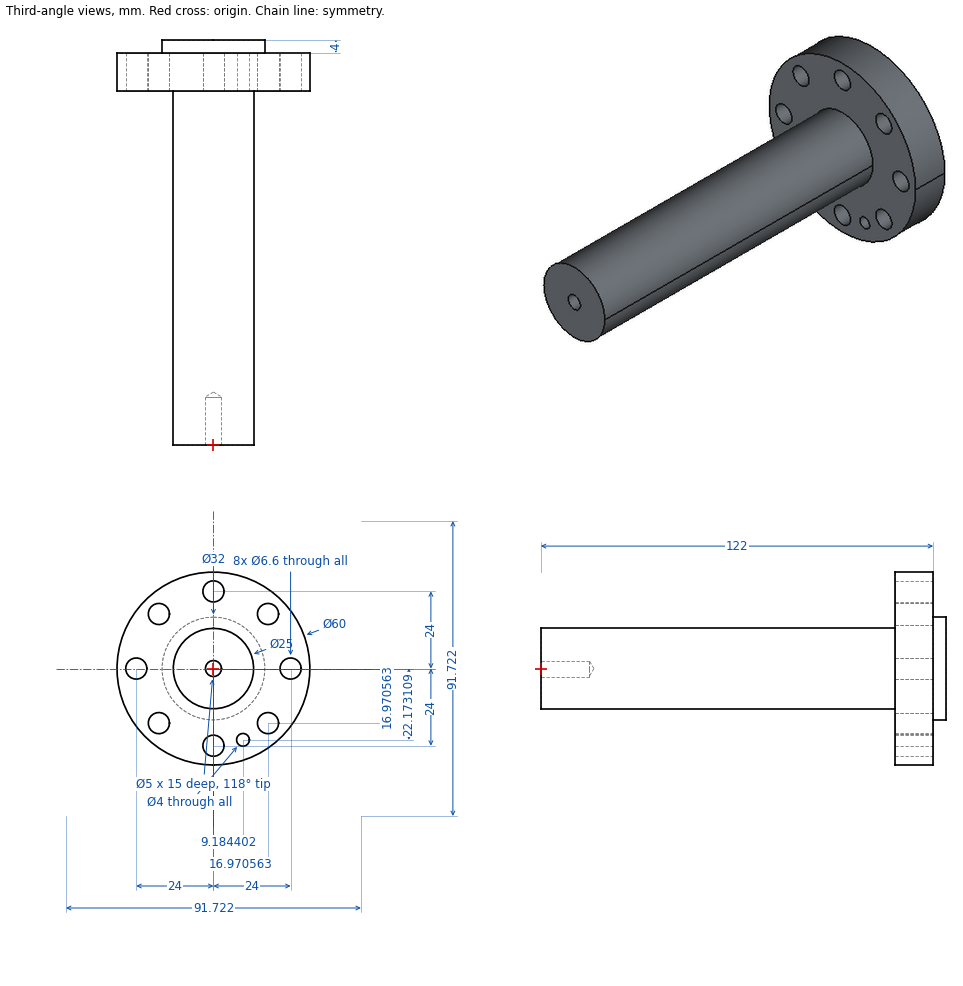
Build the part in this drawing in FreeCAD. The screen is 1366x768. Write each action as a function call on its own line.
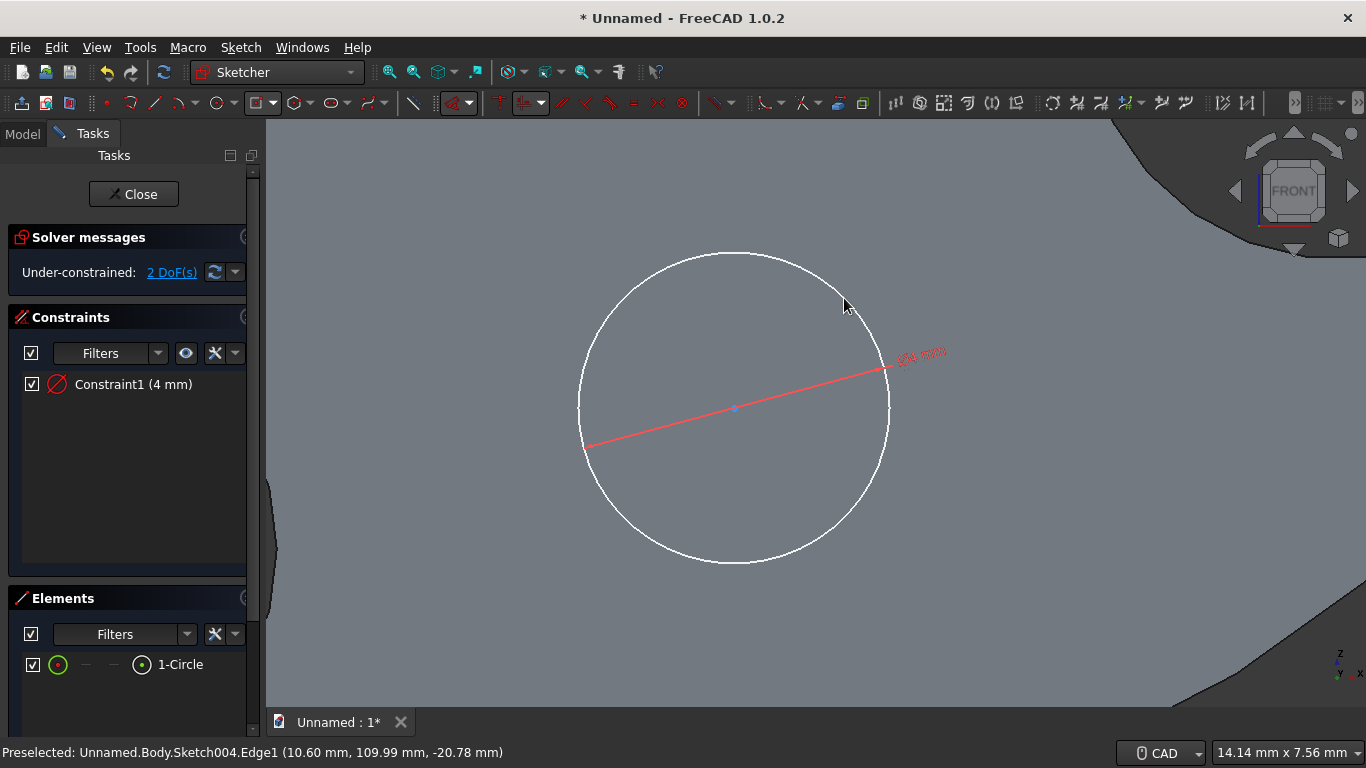
click(734, 408)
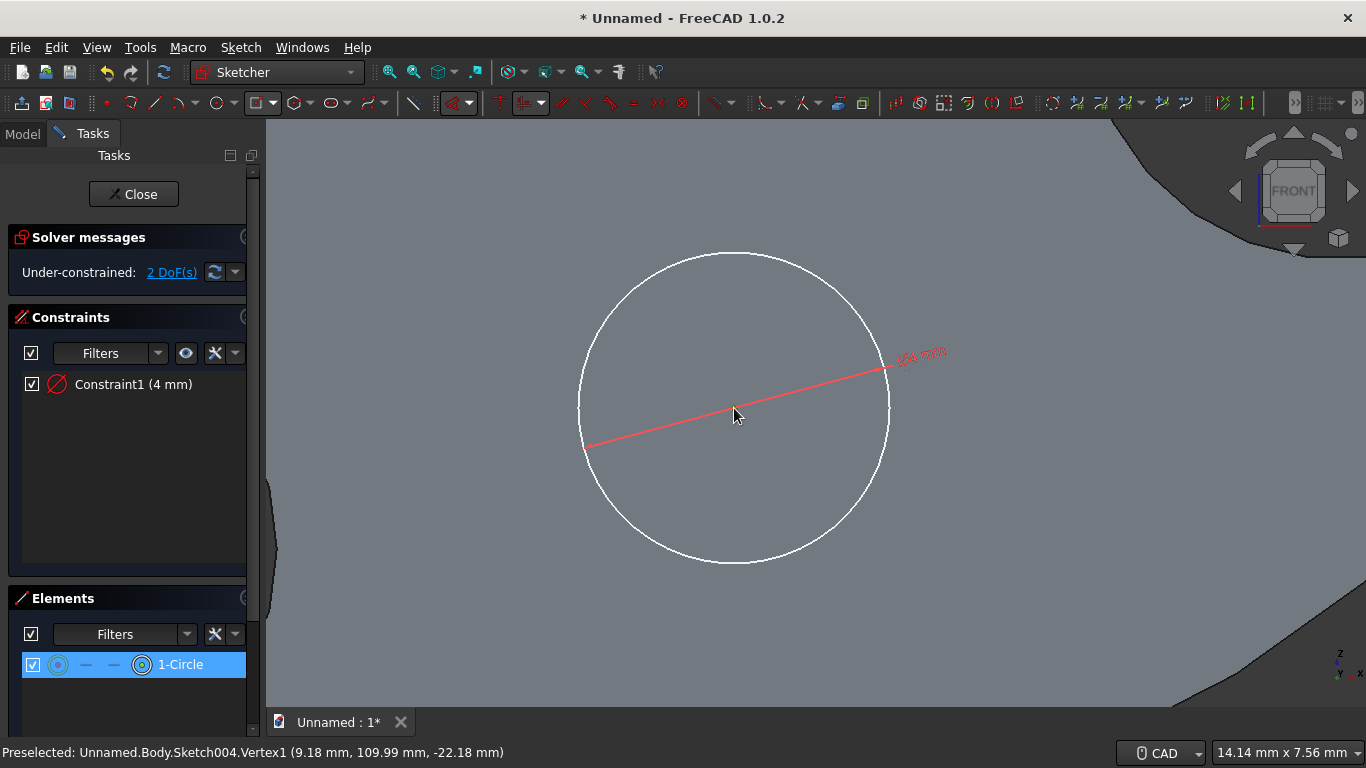
key(l)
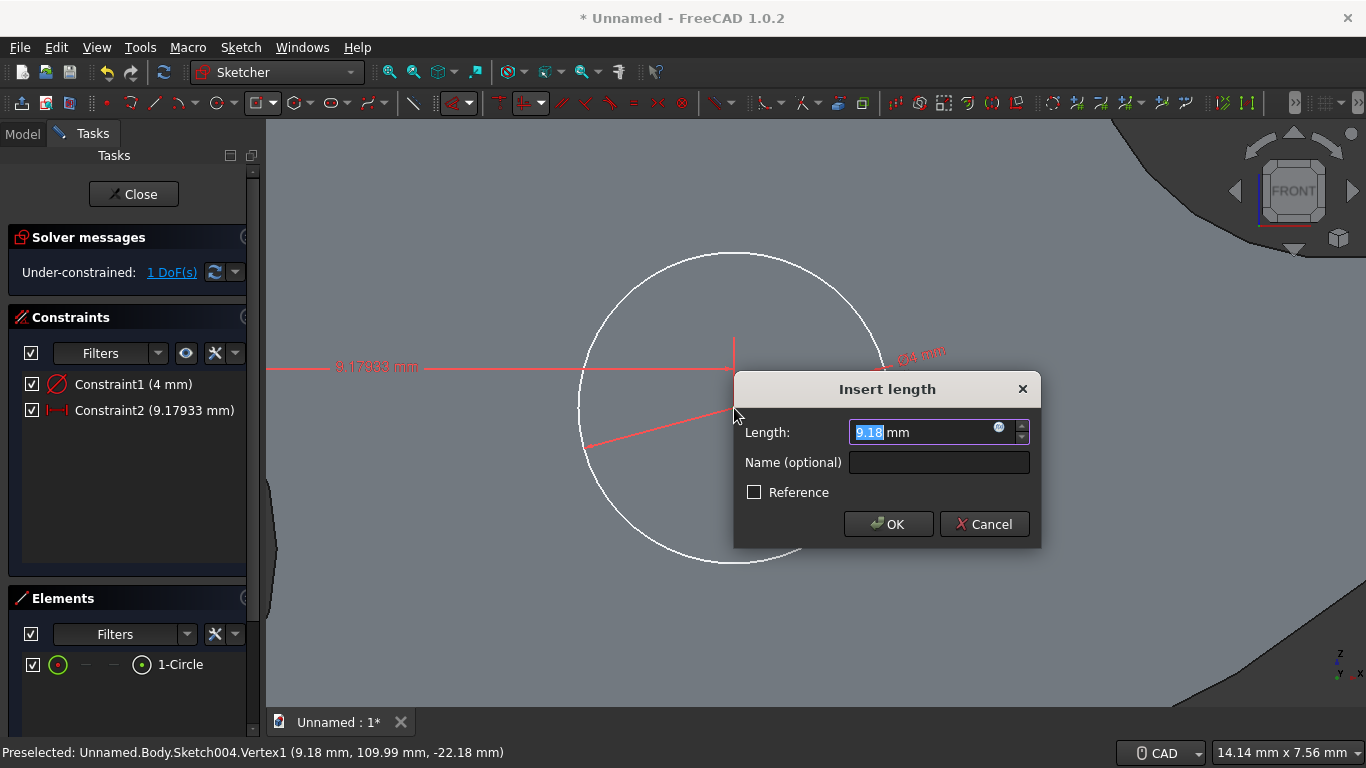
text(9.184402)
key(Return)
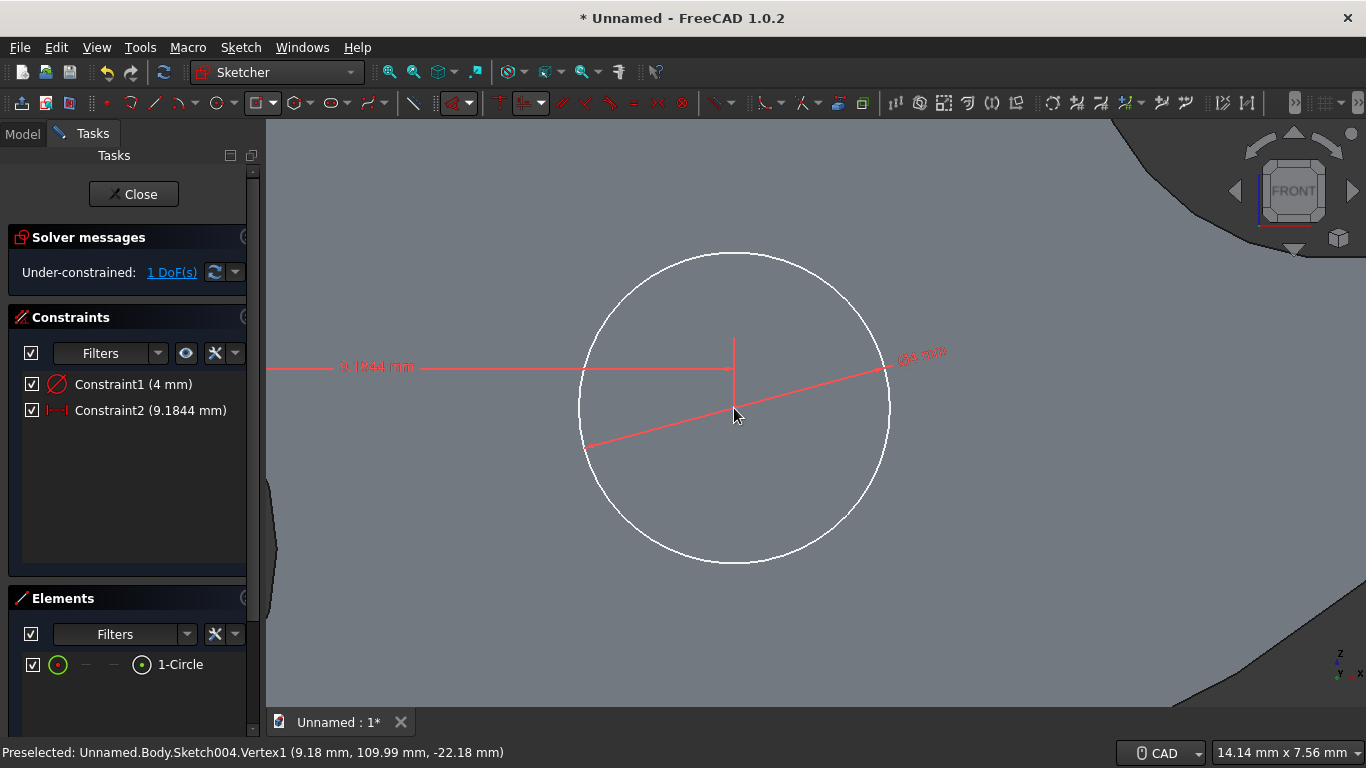
click(734, 408)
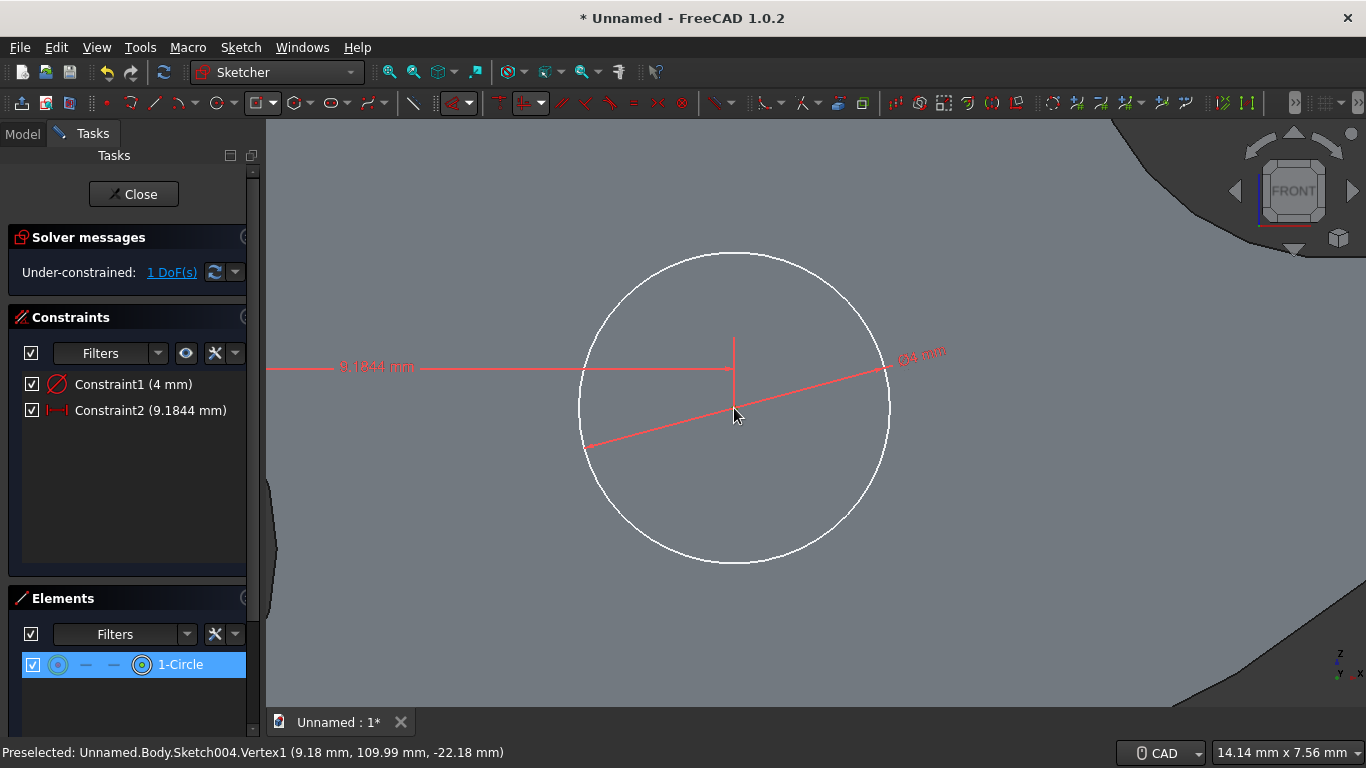
key(i)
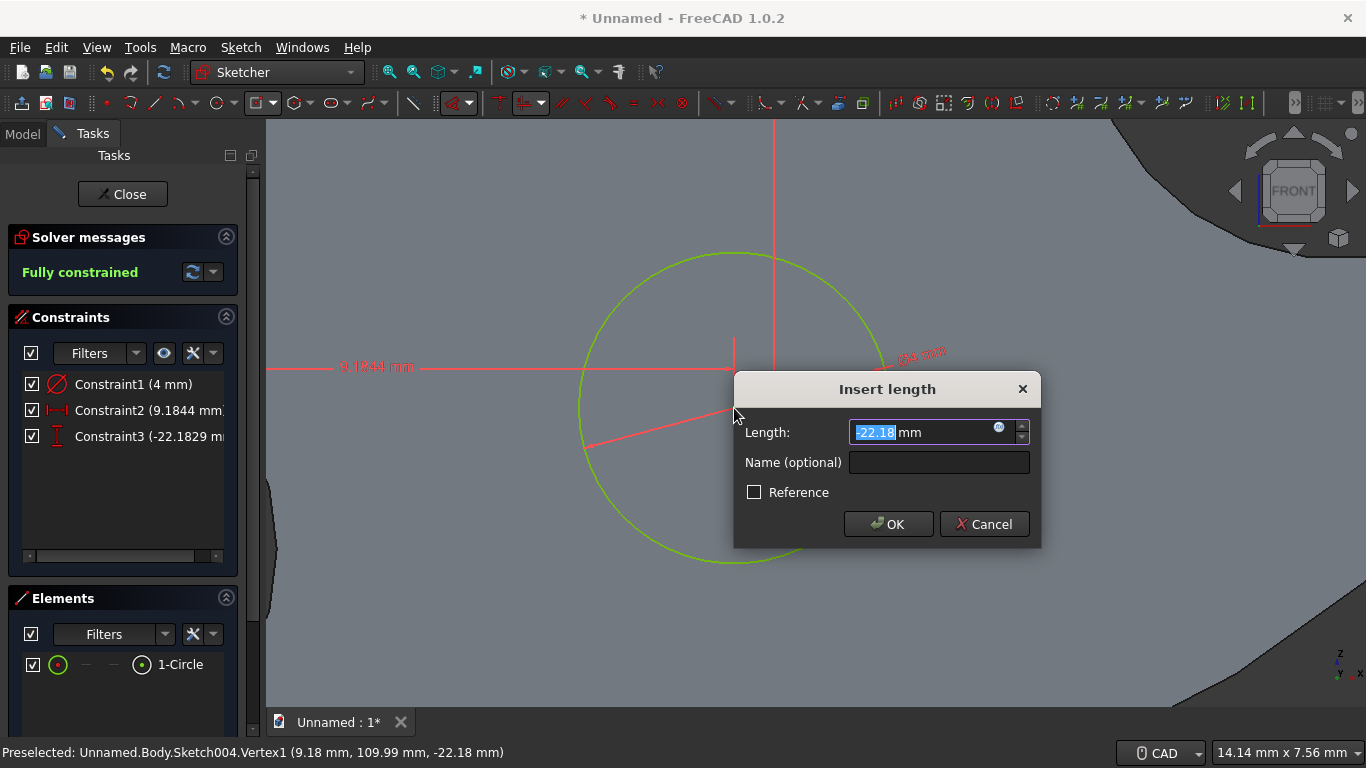
text(-22.173109)
key(Return)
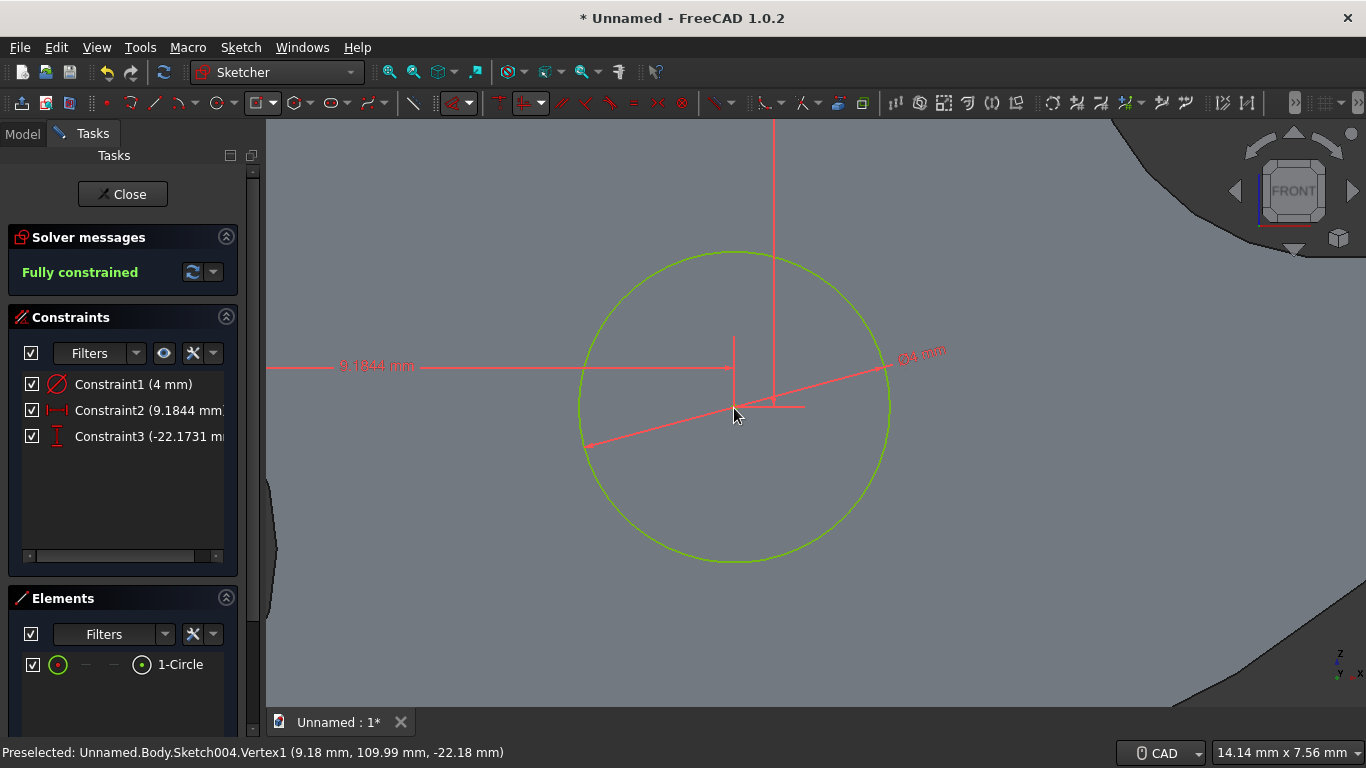
click(123, 194)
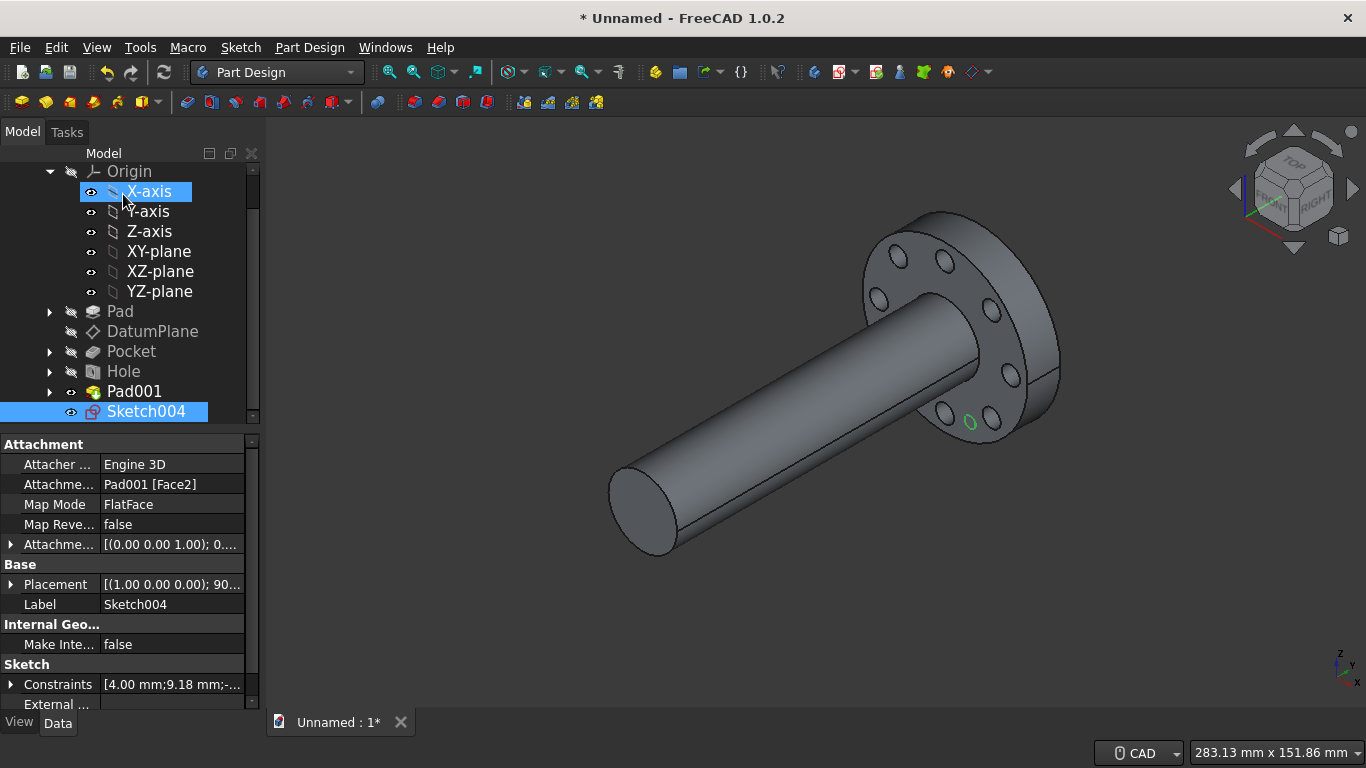
click(212, 102)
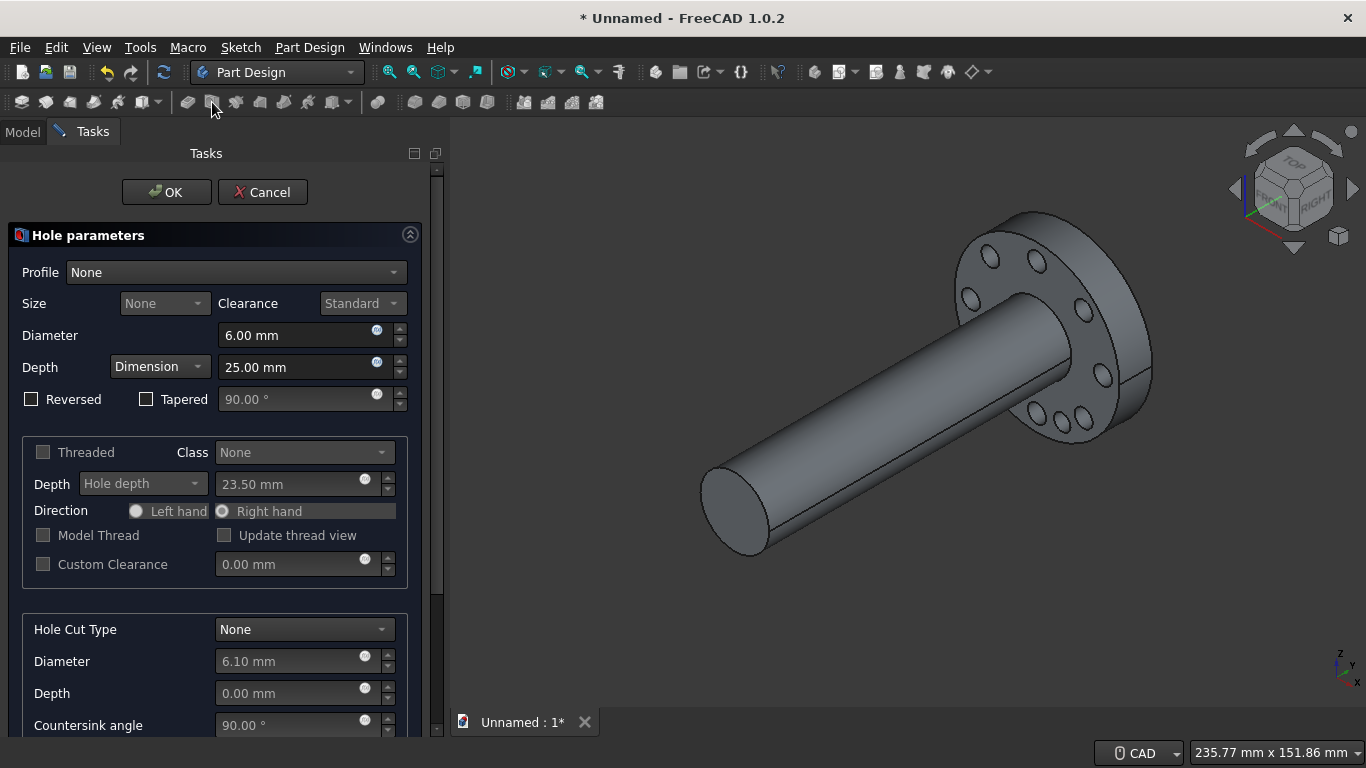
triple_click(305, 335)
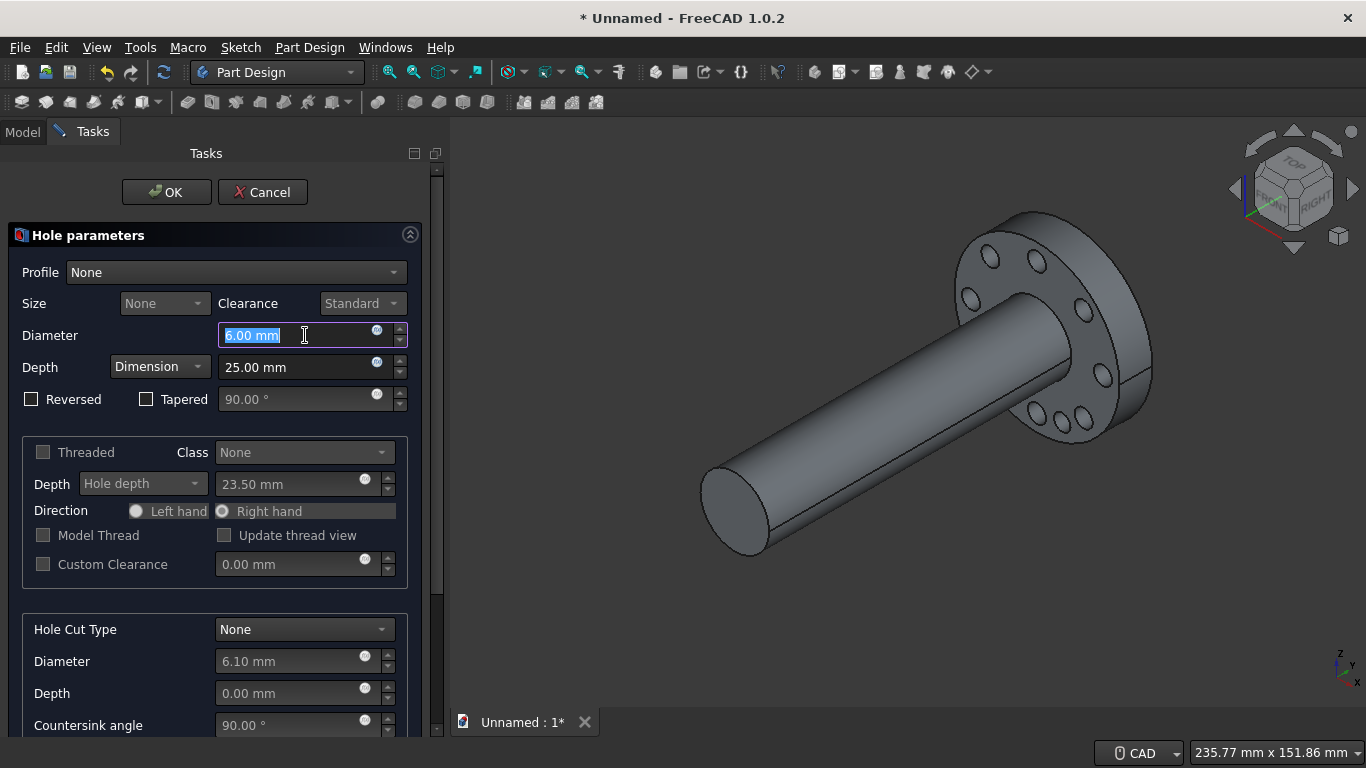
text(4)
key(Tab)